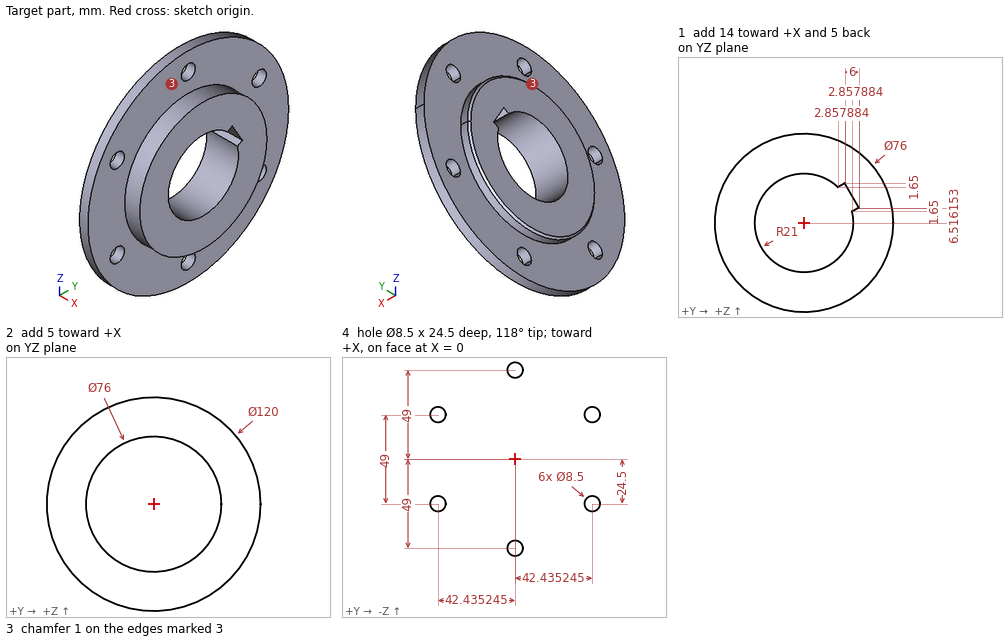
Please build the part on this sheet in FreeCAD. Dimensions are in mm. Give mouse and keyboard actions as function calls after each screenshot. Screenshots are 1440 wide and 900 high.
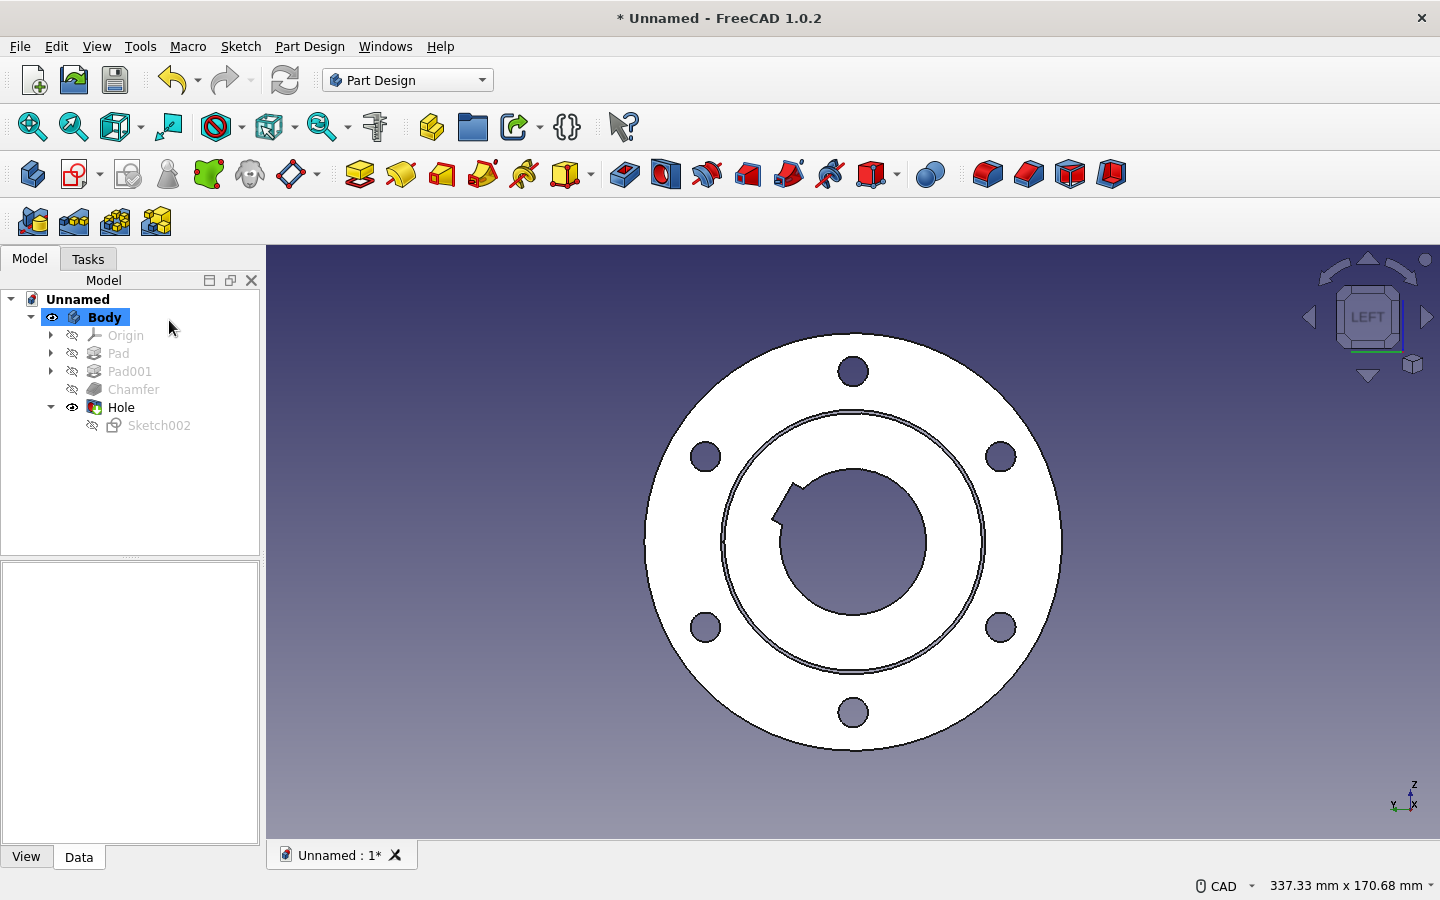
key(0)